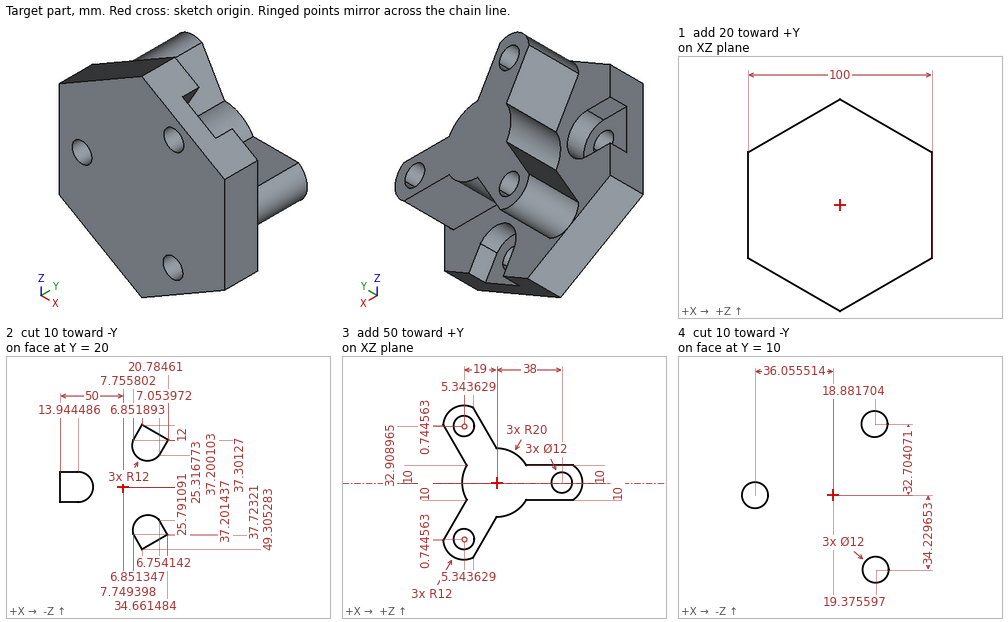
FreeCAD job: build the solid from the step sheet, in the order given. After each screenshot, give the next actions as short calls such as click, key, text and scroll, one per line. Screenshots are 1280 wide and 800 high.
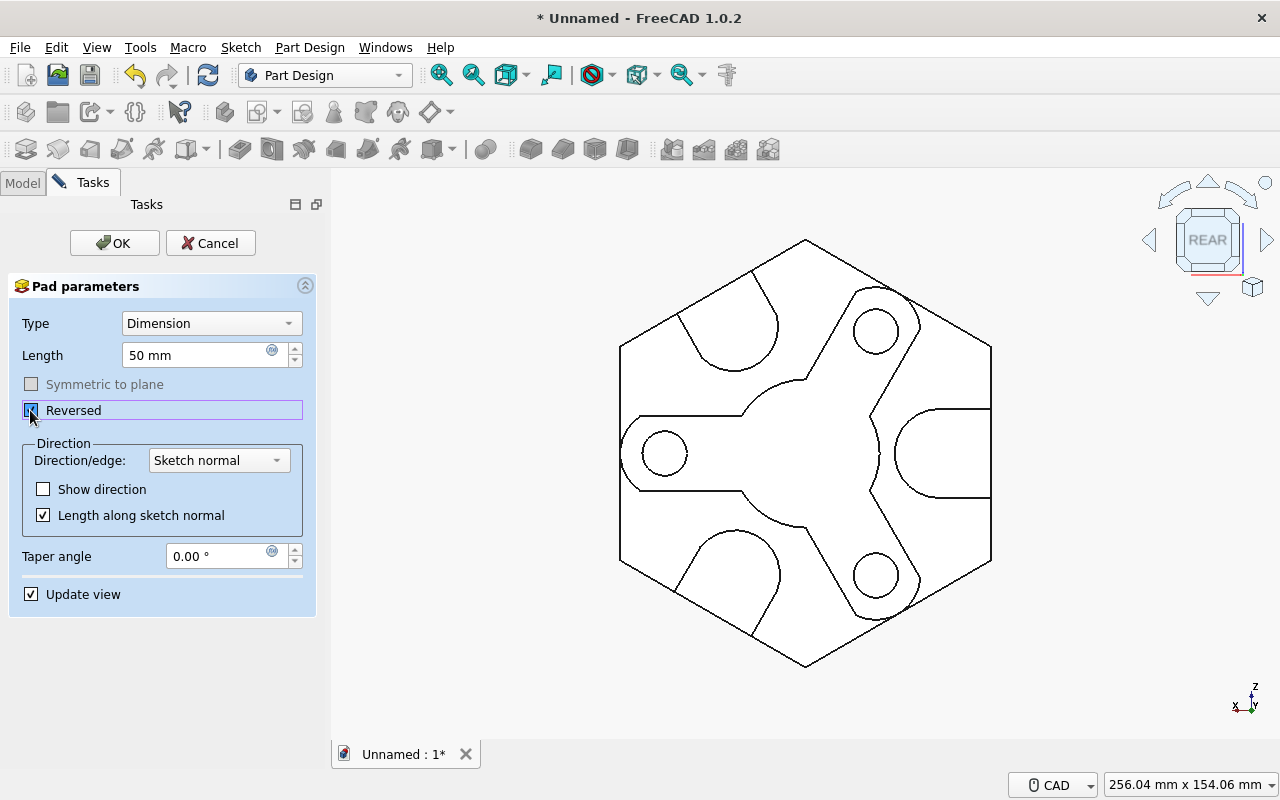
click(115, 243)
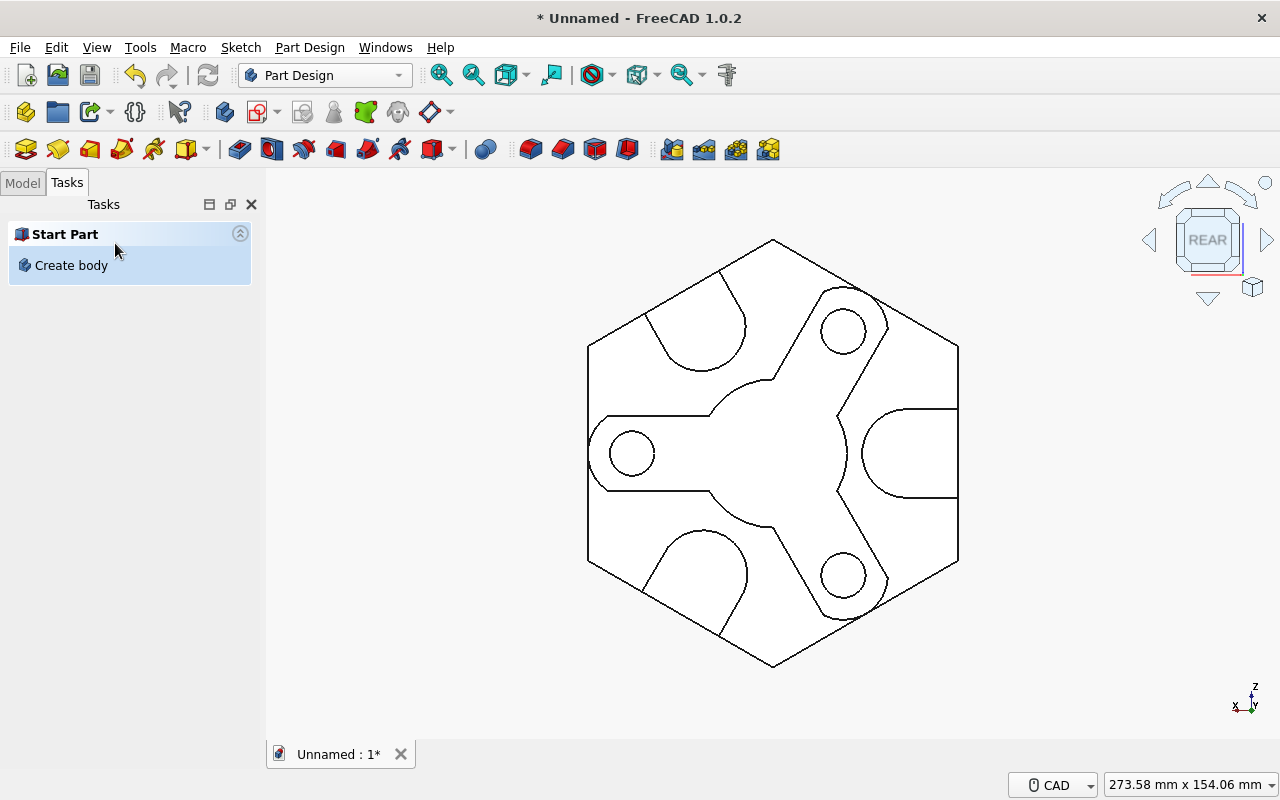
click(910, 453)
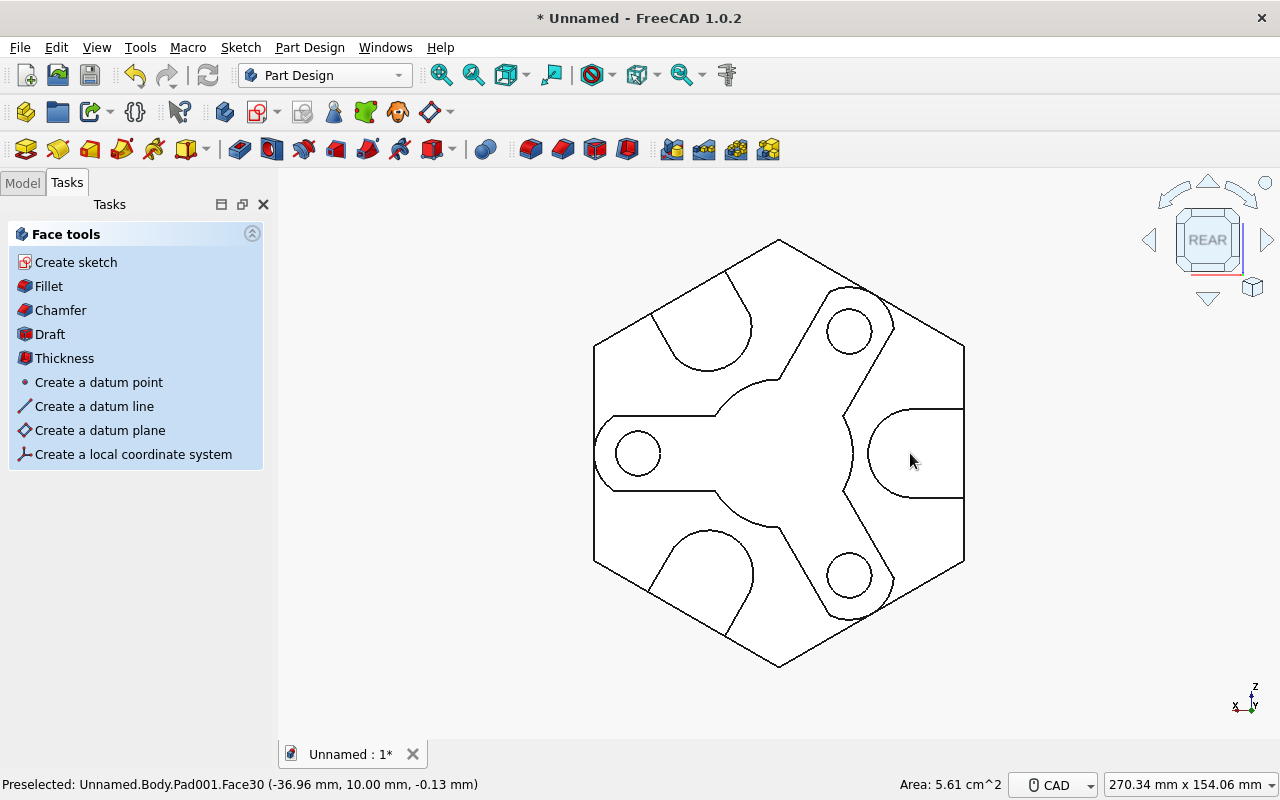
click(258, 112)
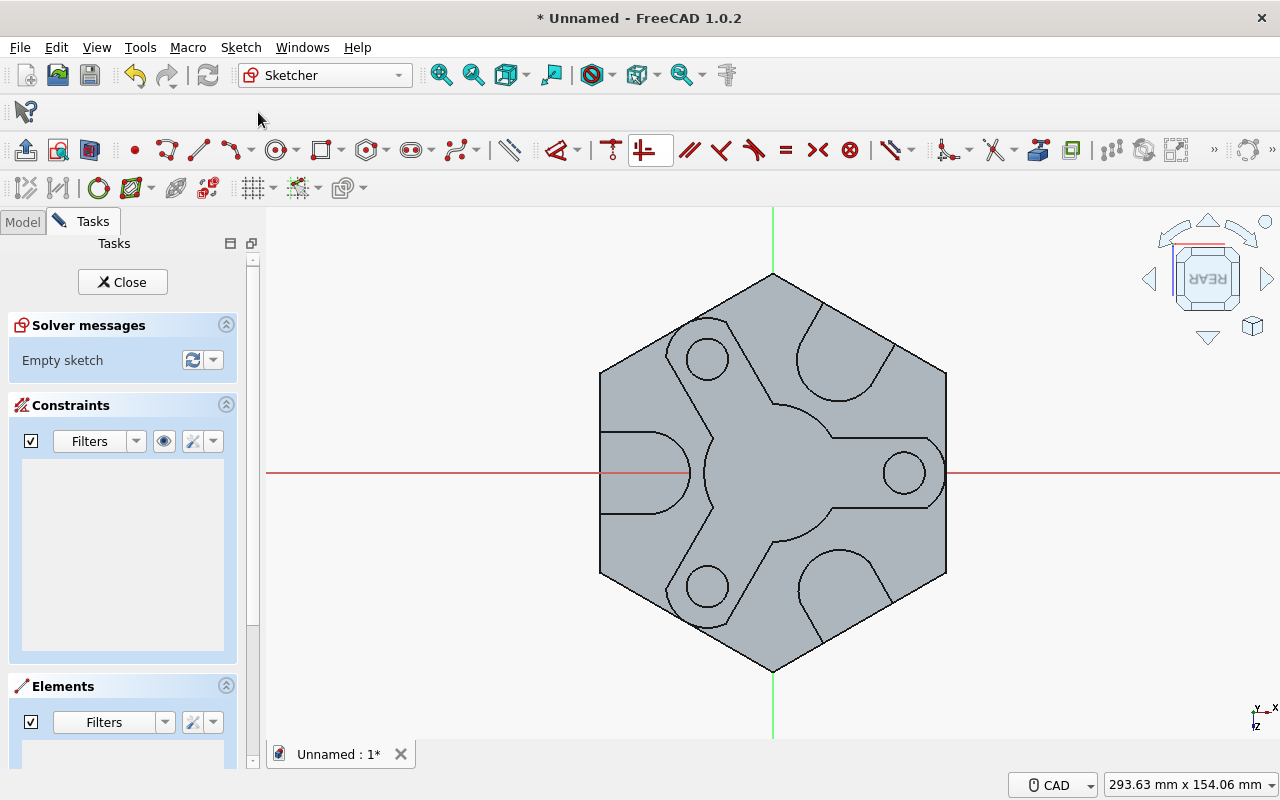
click(90, 150)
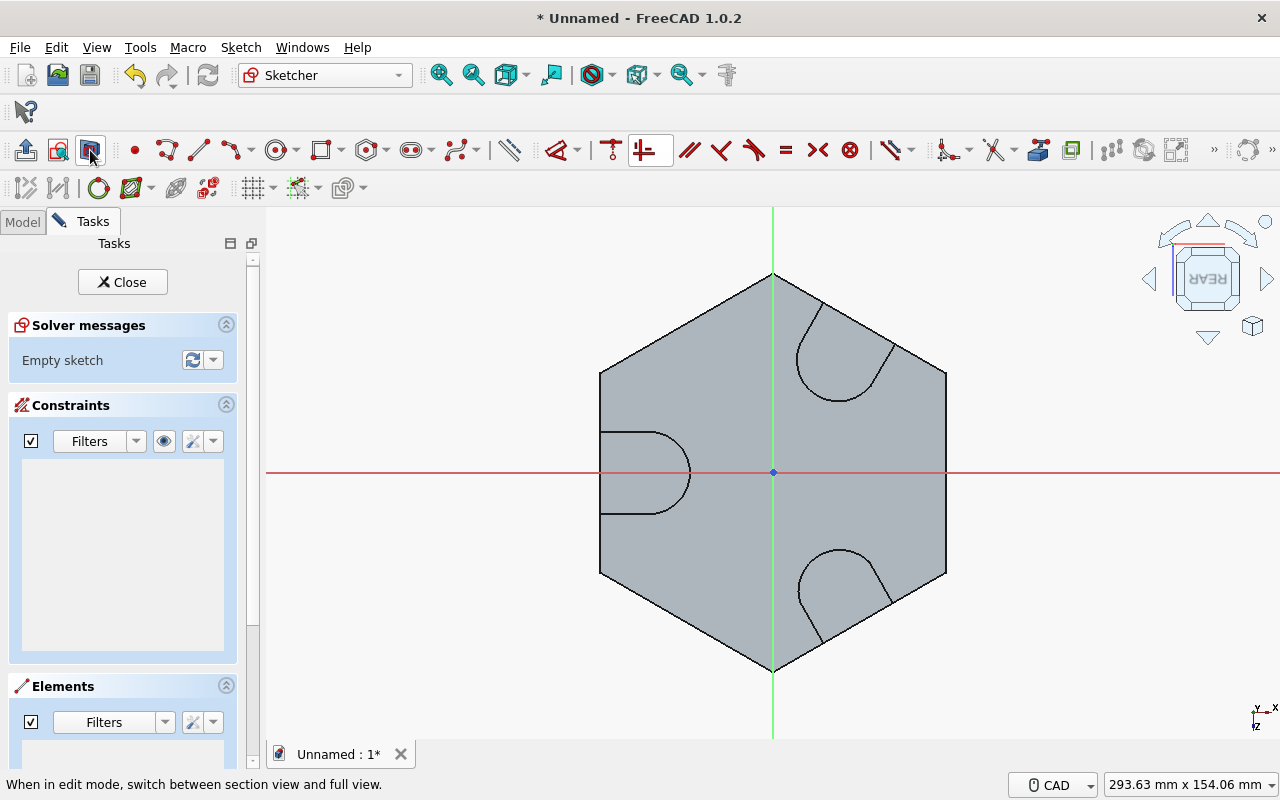
click(276, 150)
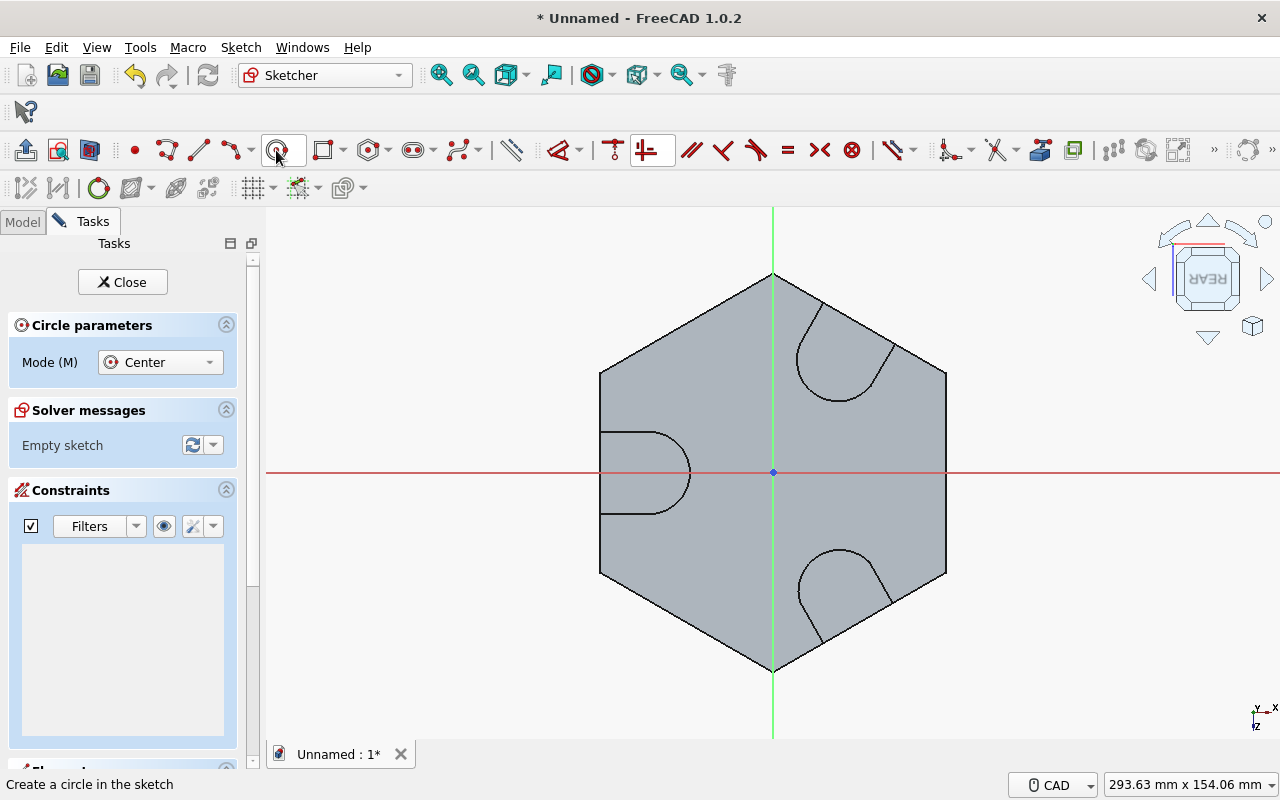
click(840, 591)
move(855, 577)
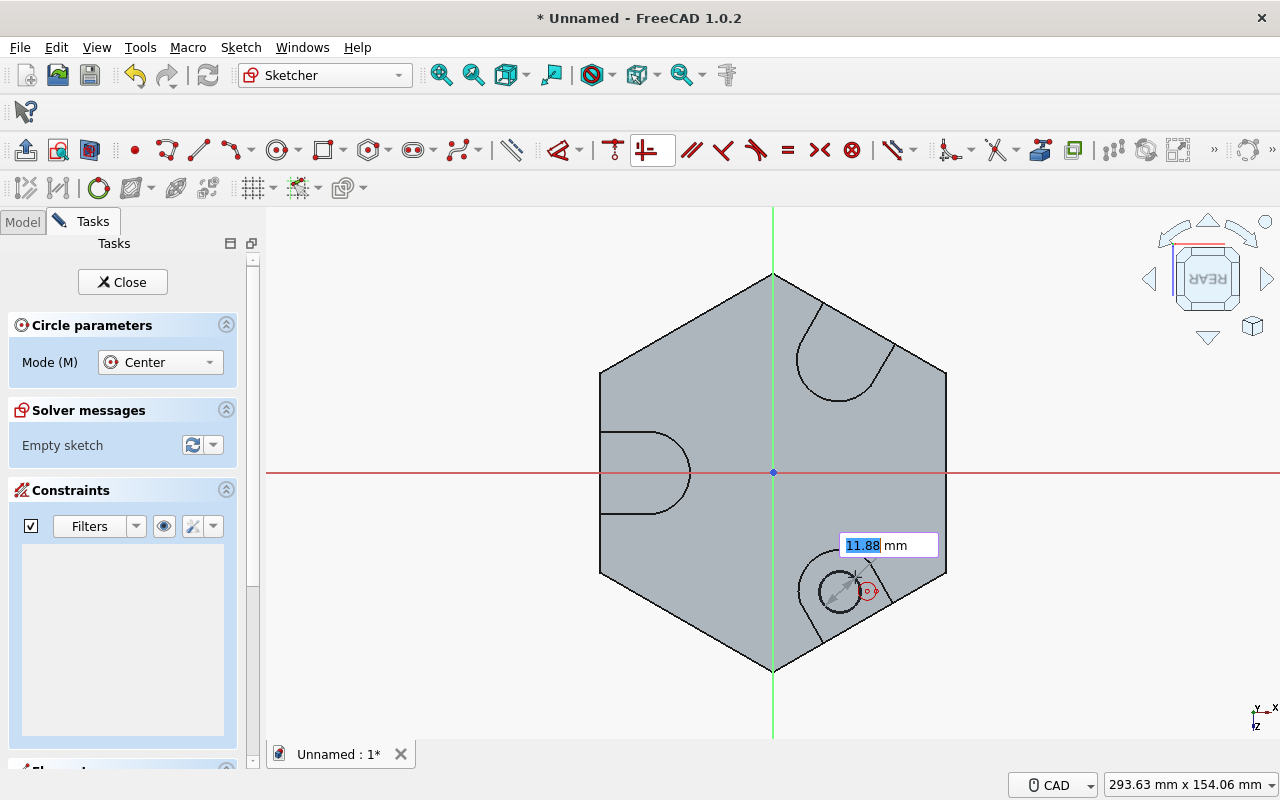
text(12)
key(Return)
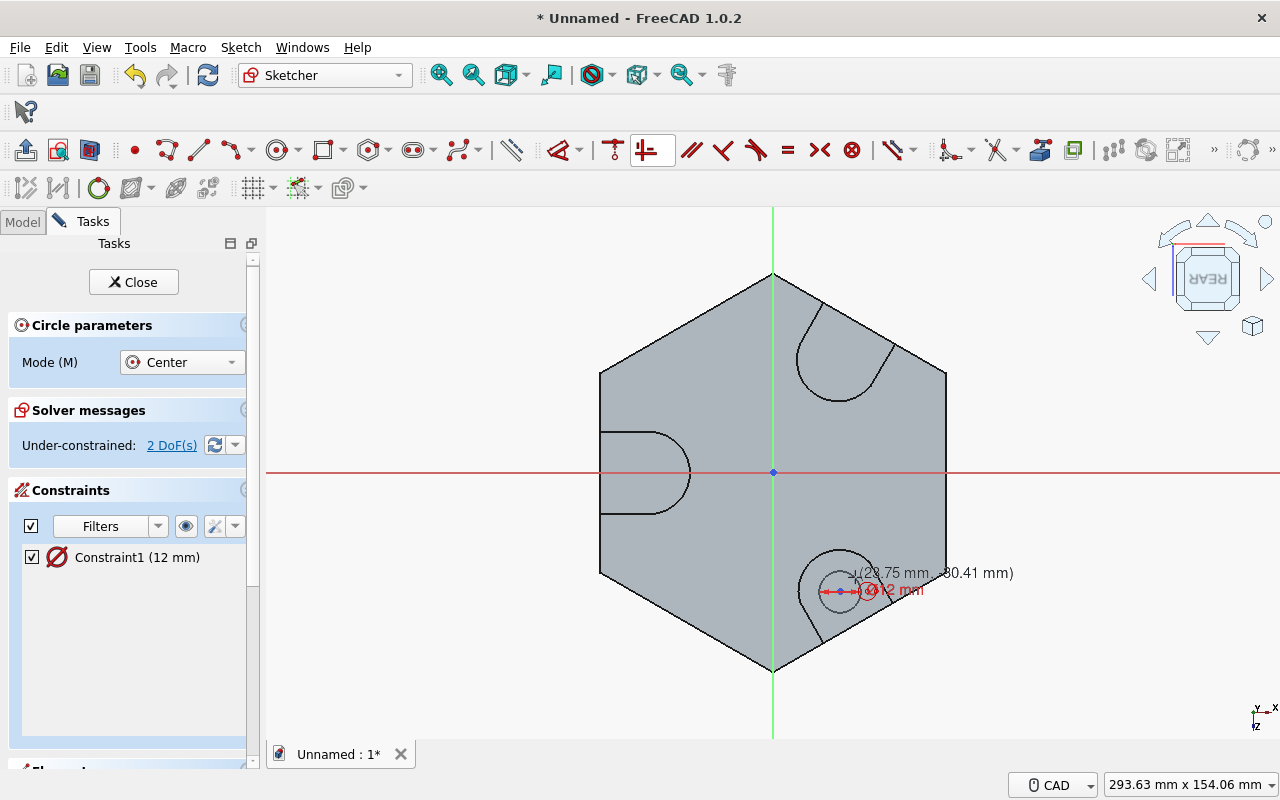
click(648, 473)
move(663, 458)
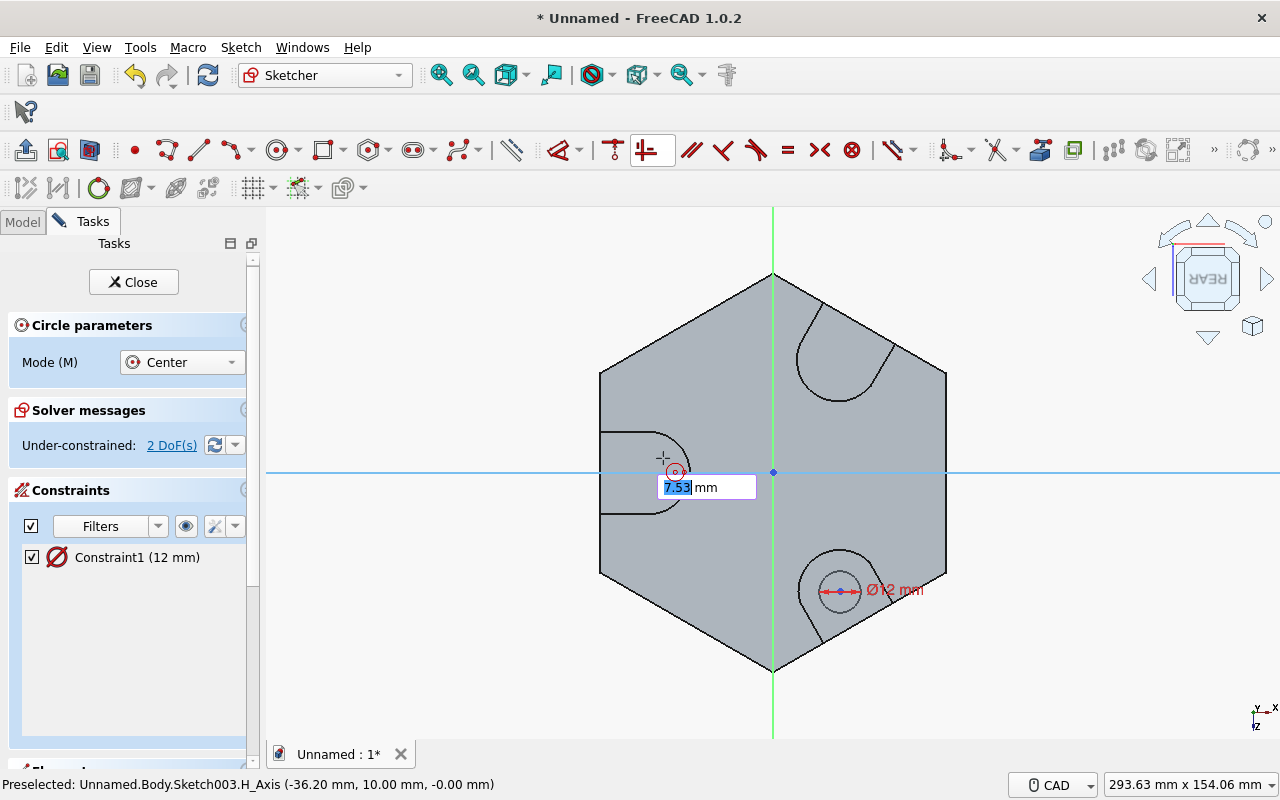
text(12)
key(Return)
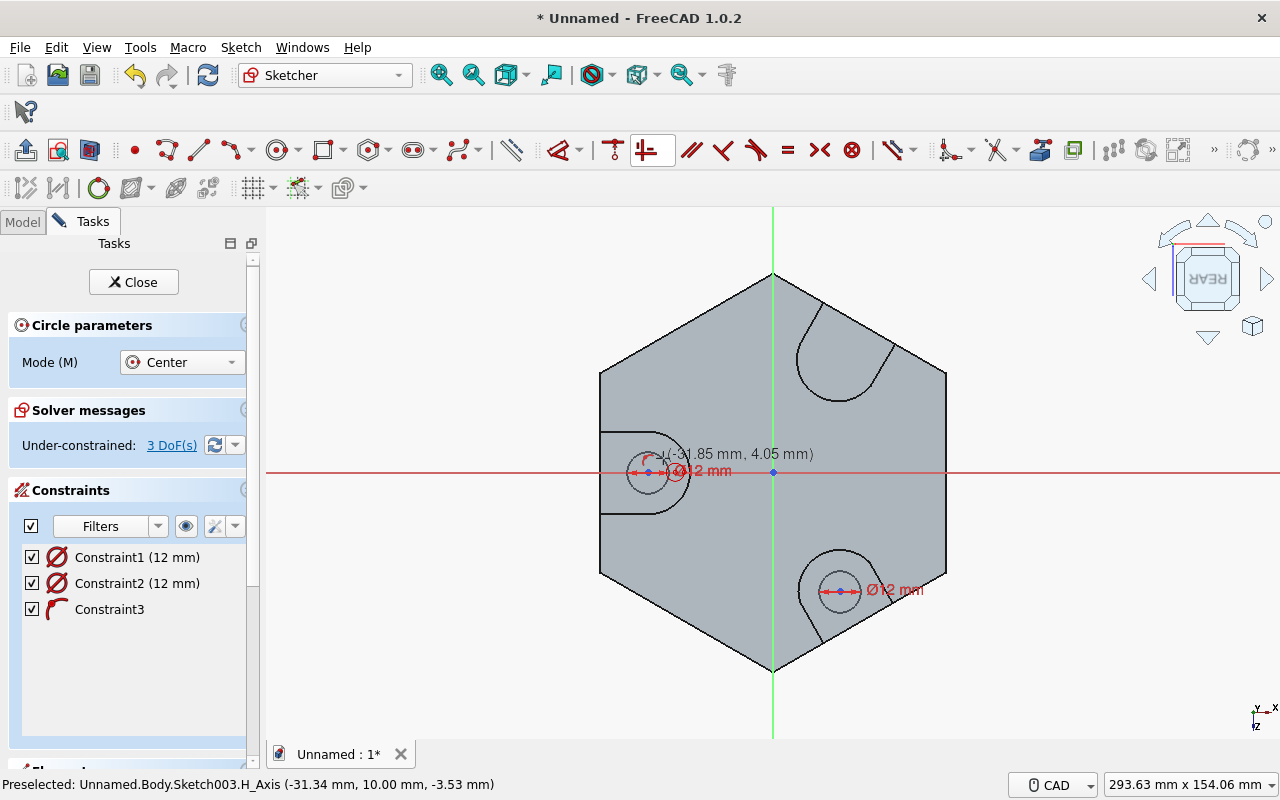
click(838, 360)
move(853, 345)